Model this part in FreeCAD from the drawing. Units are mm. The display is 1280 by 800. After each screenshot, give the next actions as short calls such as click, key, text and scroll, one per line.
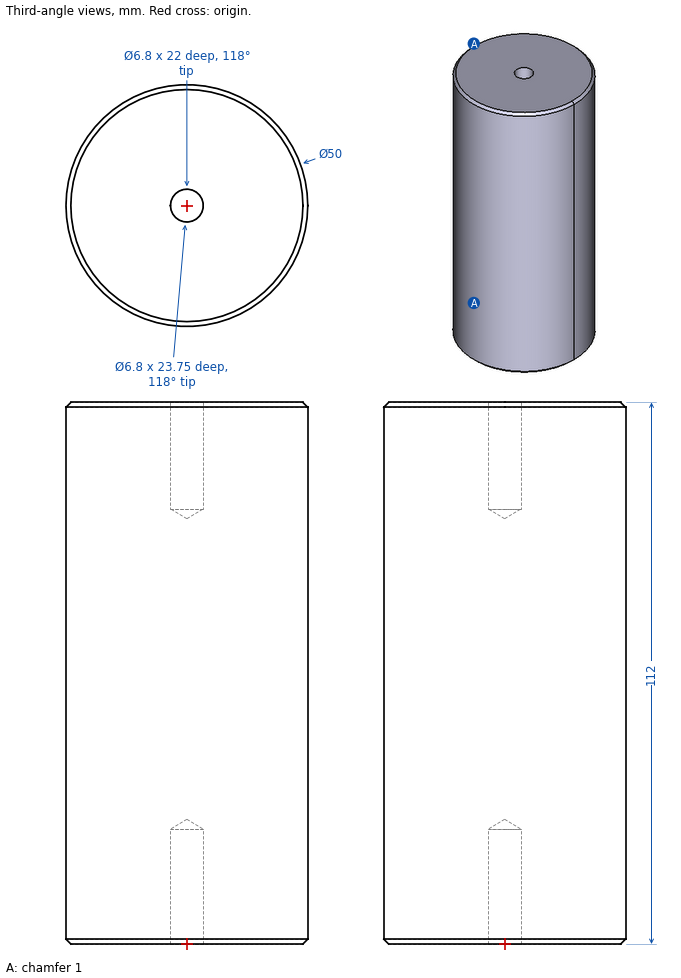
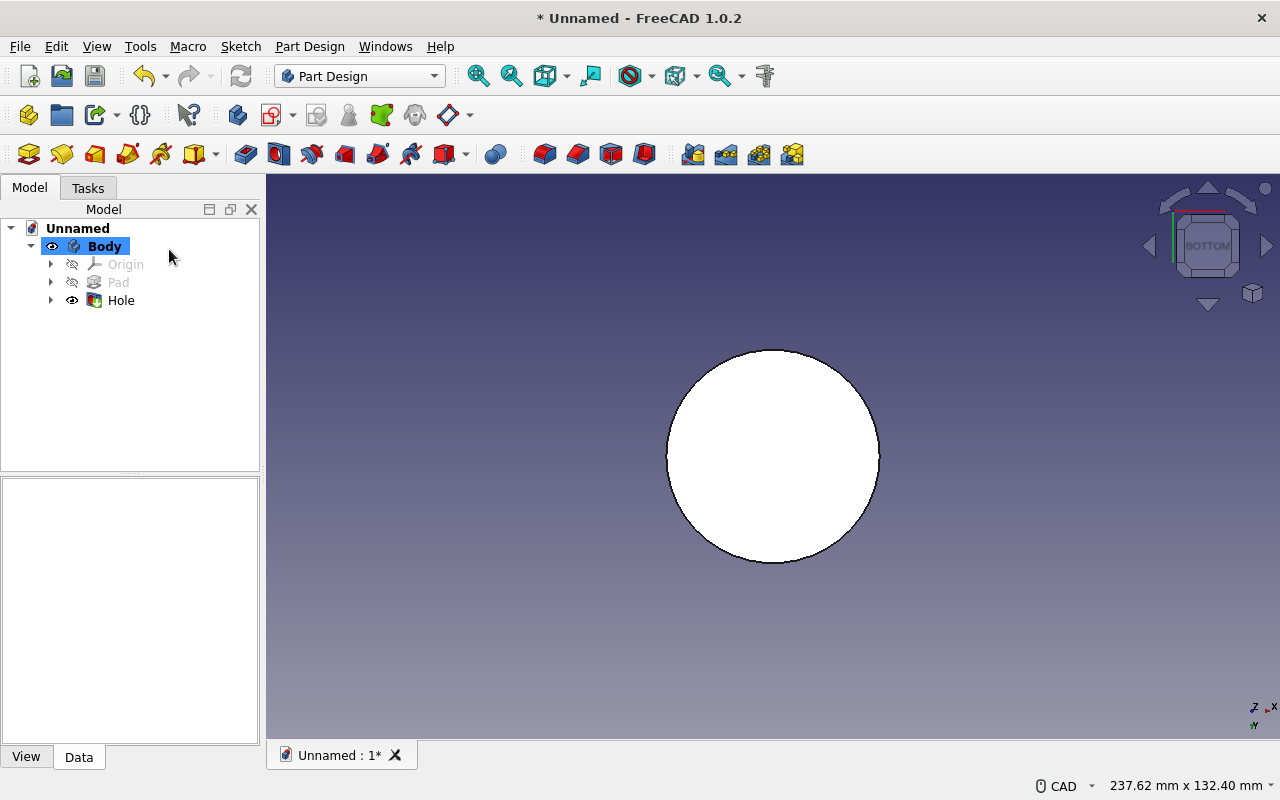
key(v)
key(f)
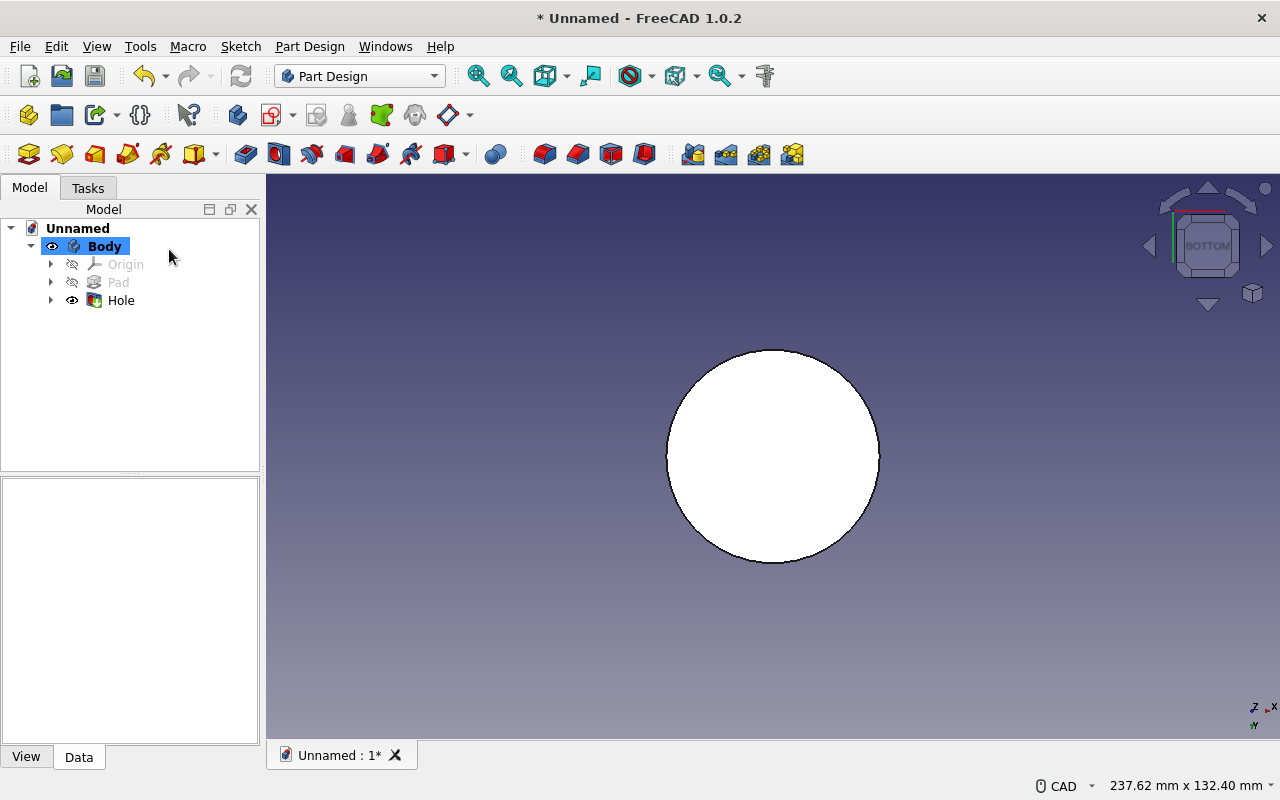
click(773, 455)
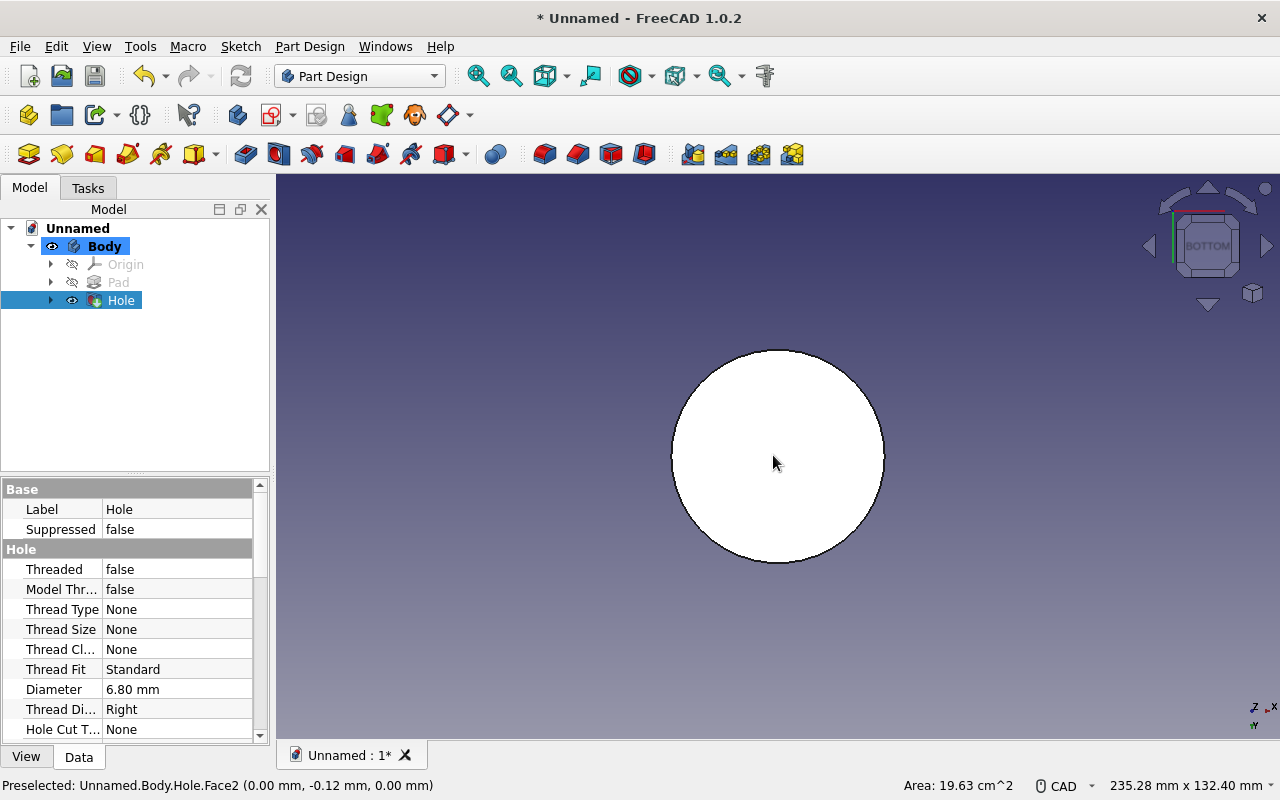
click(270, 116)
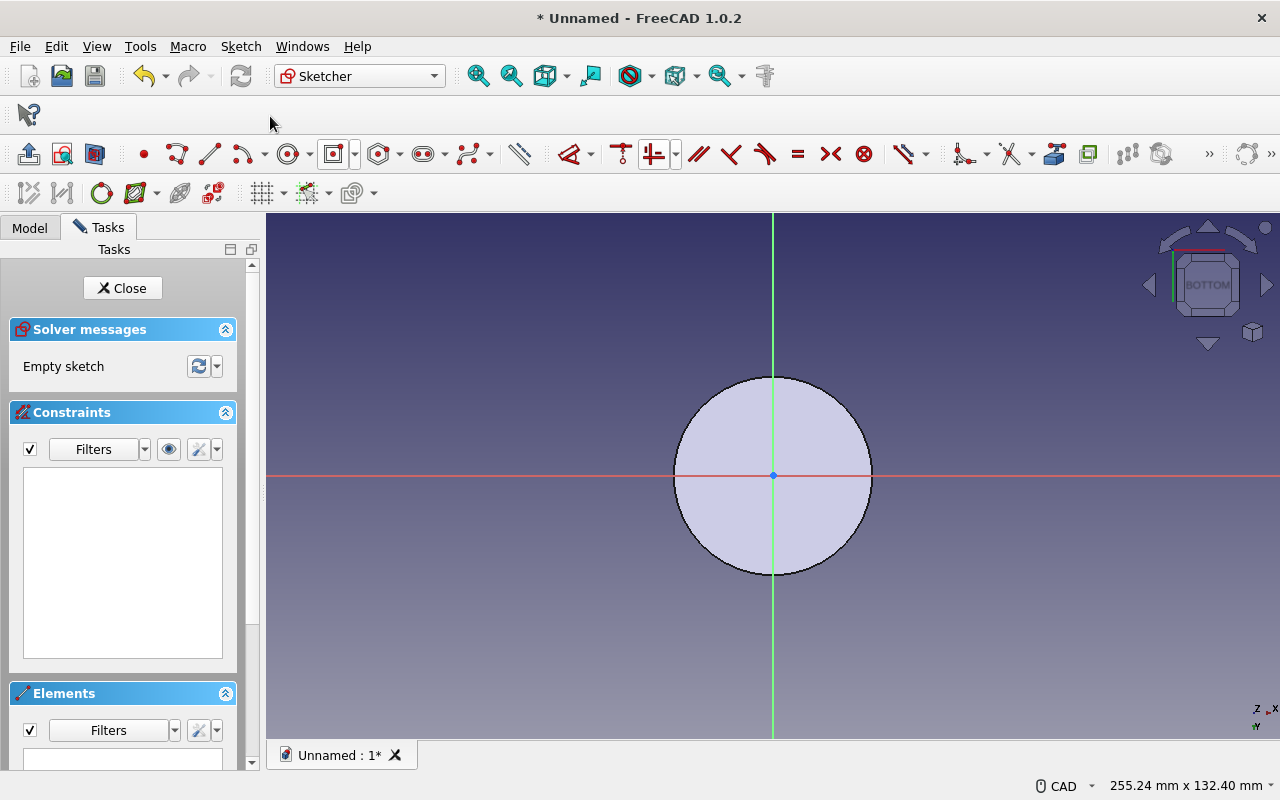
scroll(778, 476, up, 13)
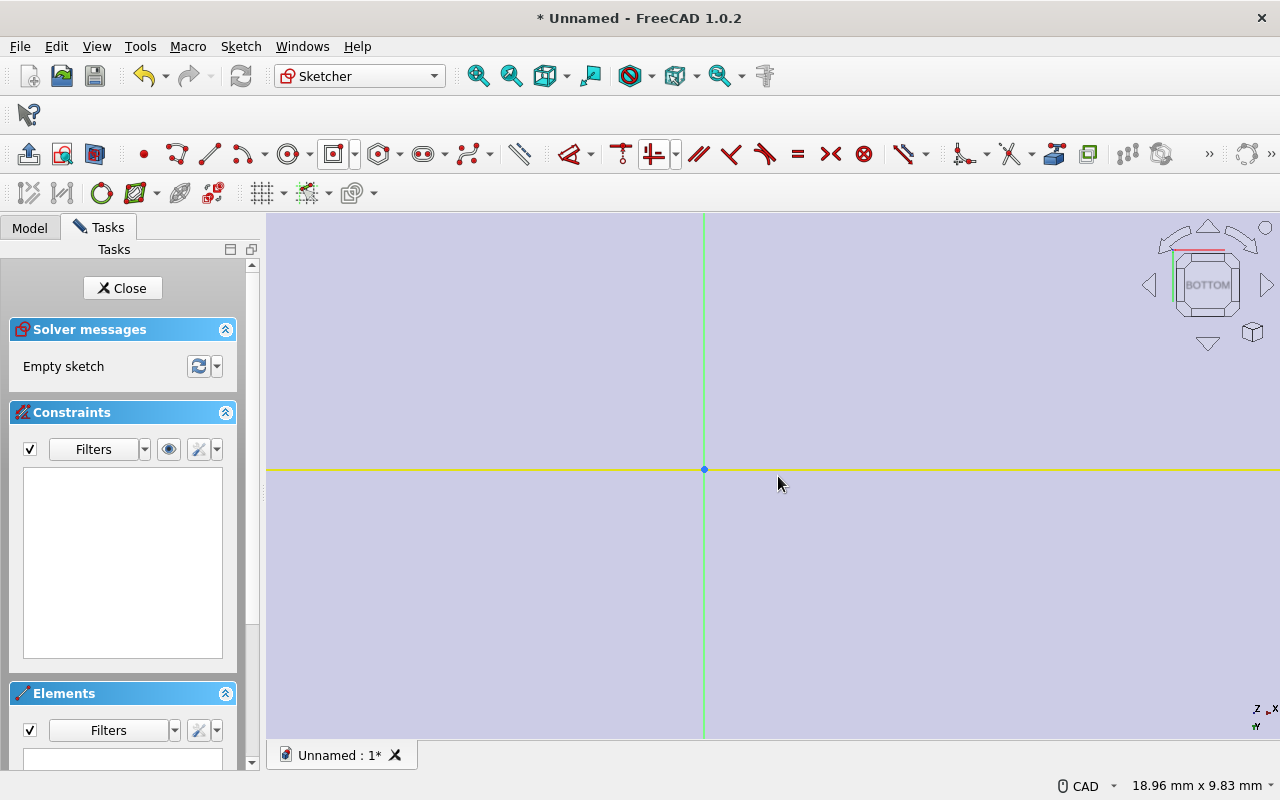
key(g)
key(c)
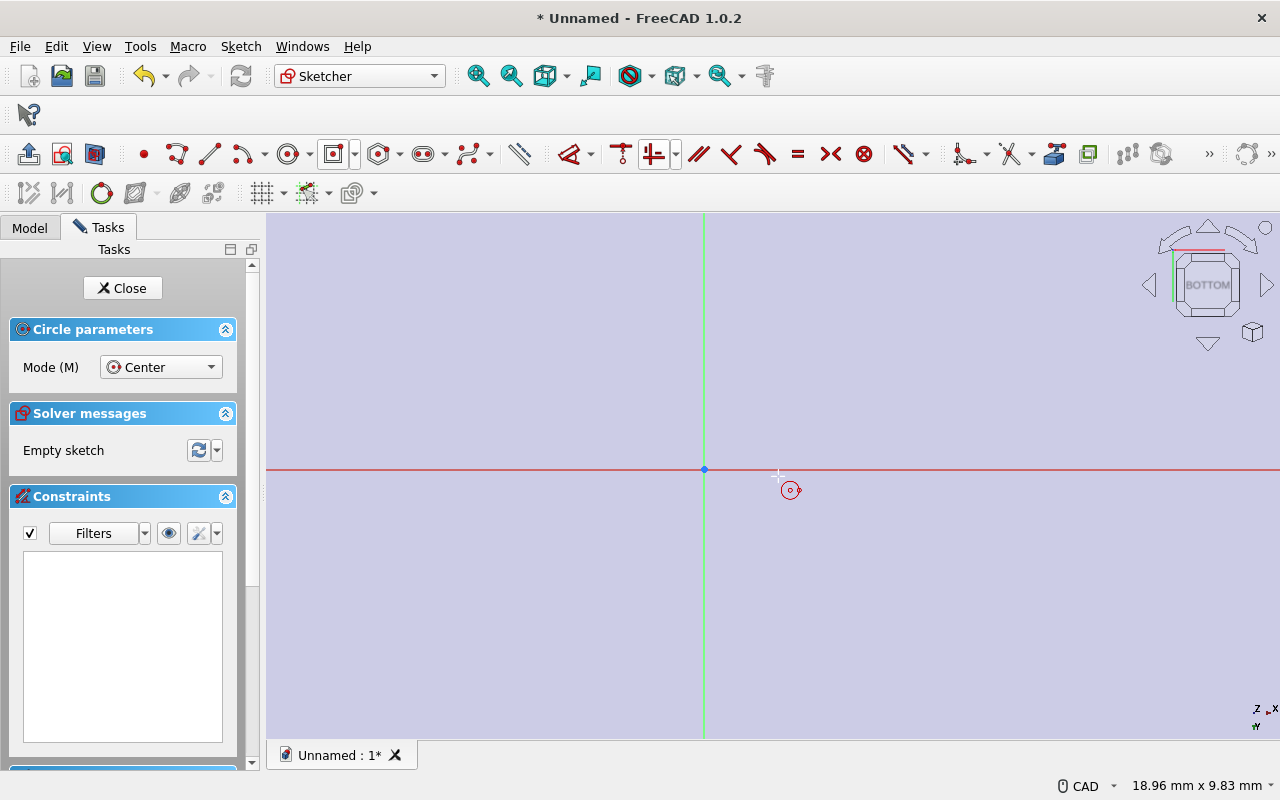
click(704, 470)
click(833, 341)
key(Escape)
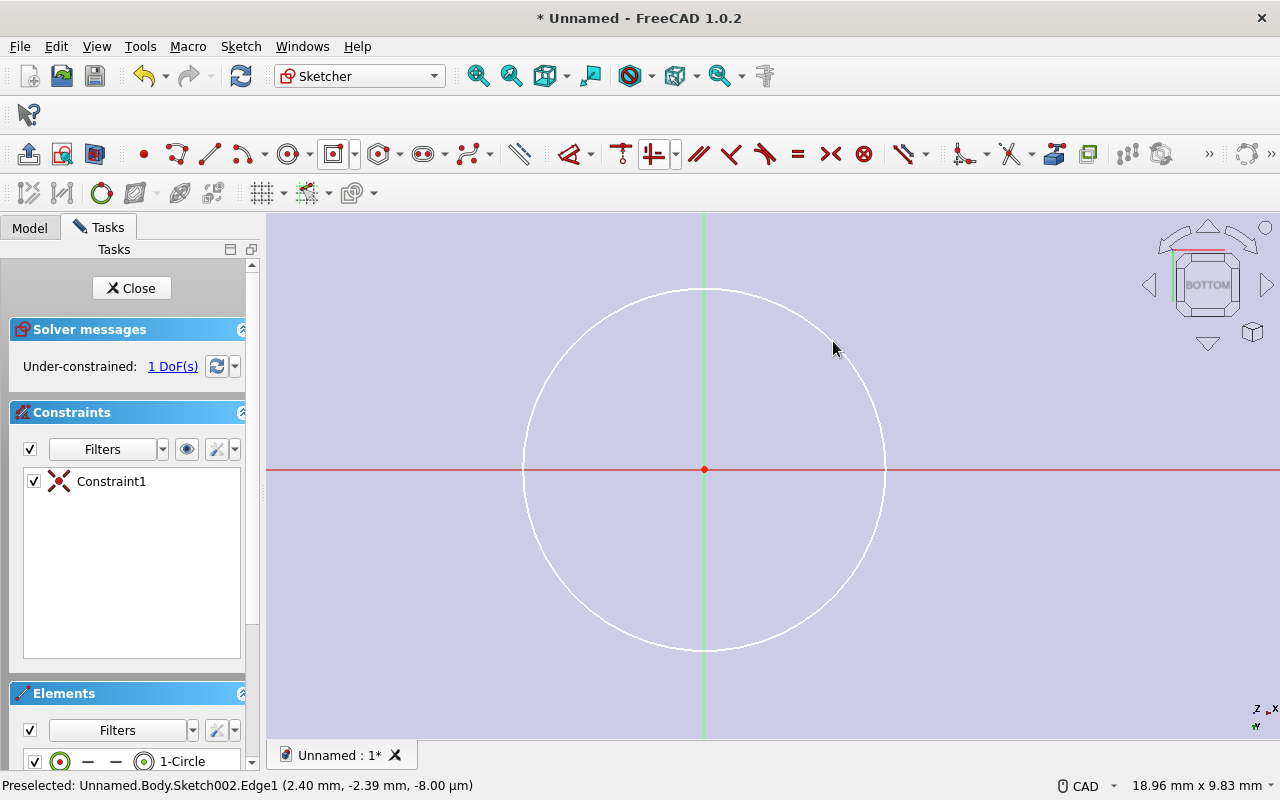
key(d)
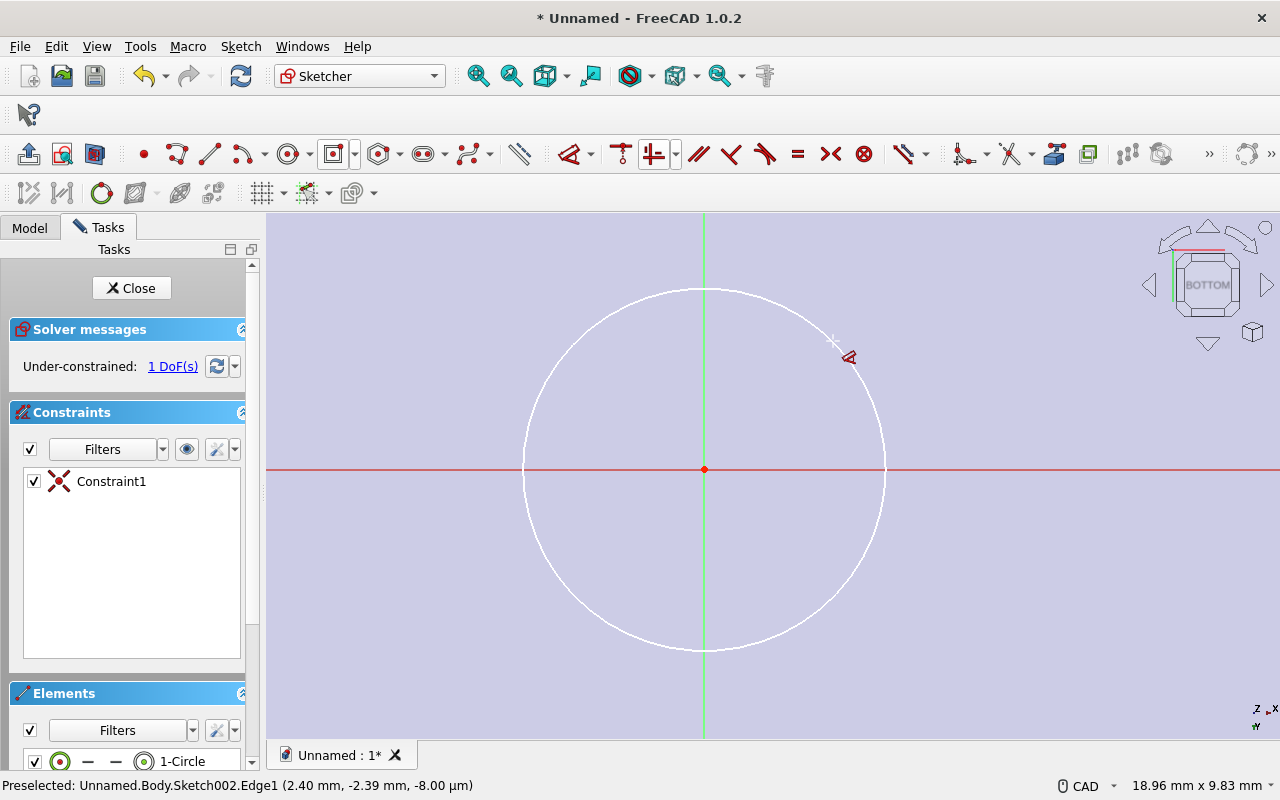
click(832, 341)
click(855, 318)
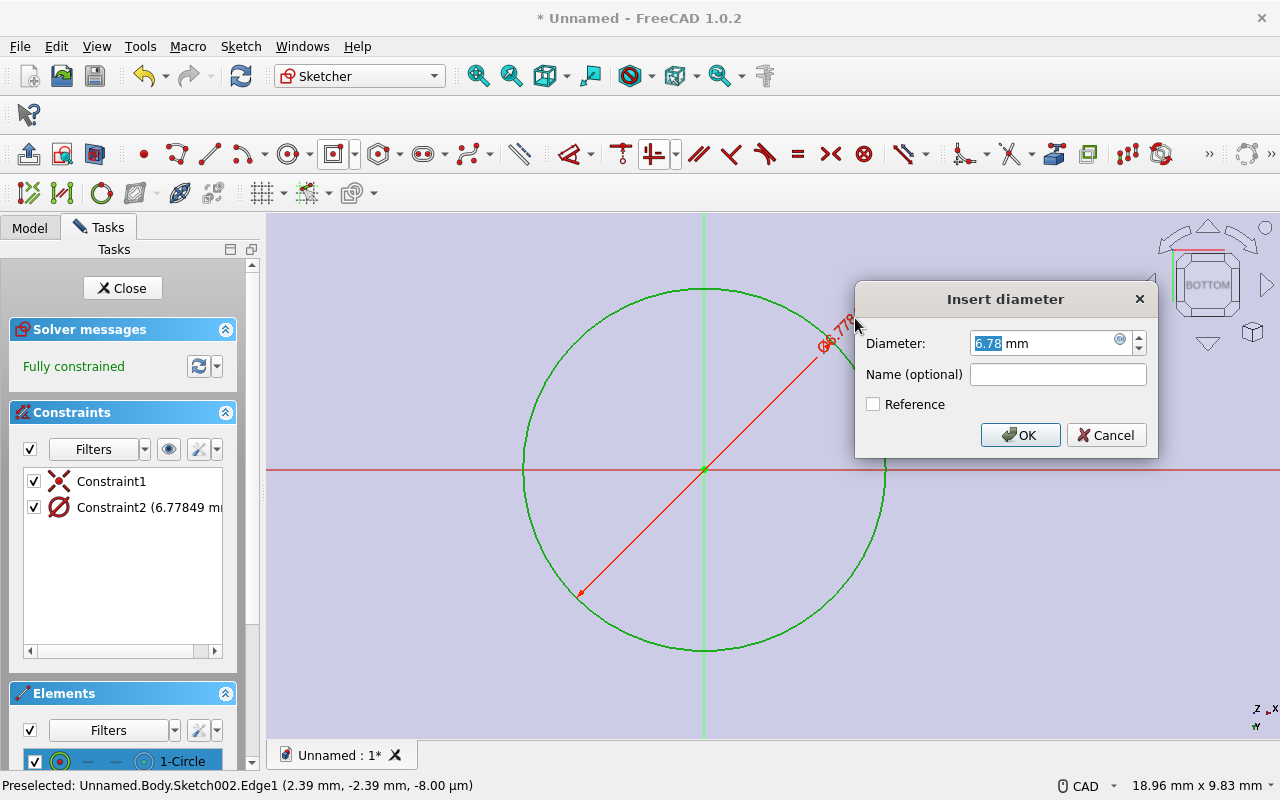
text(6.8)
key(Return)
key(Escape)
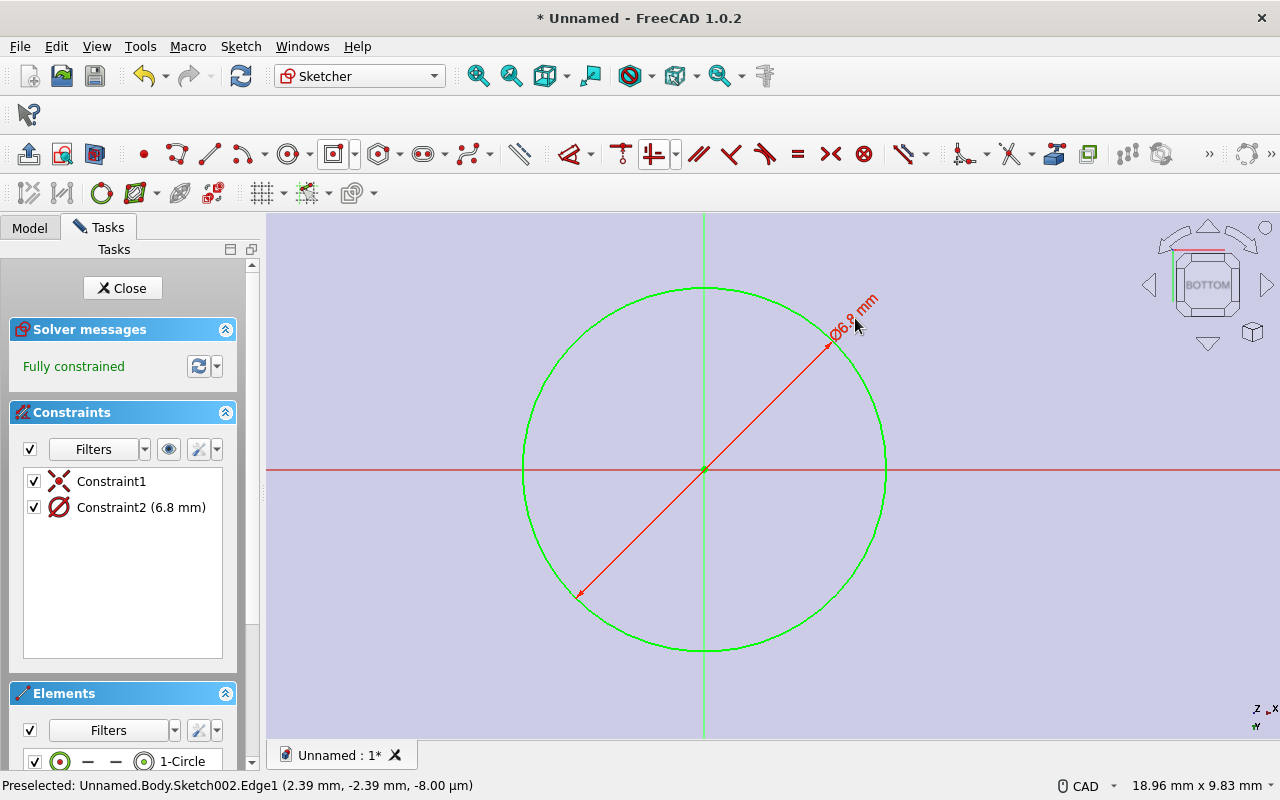
click(123, 288)